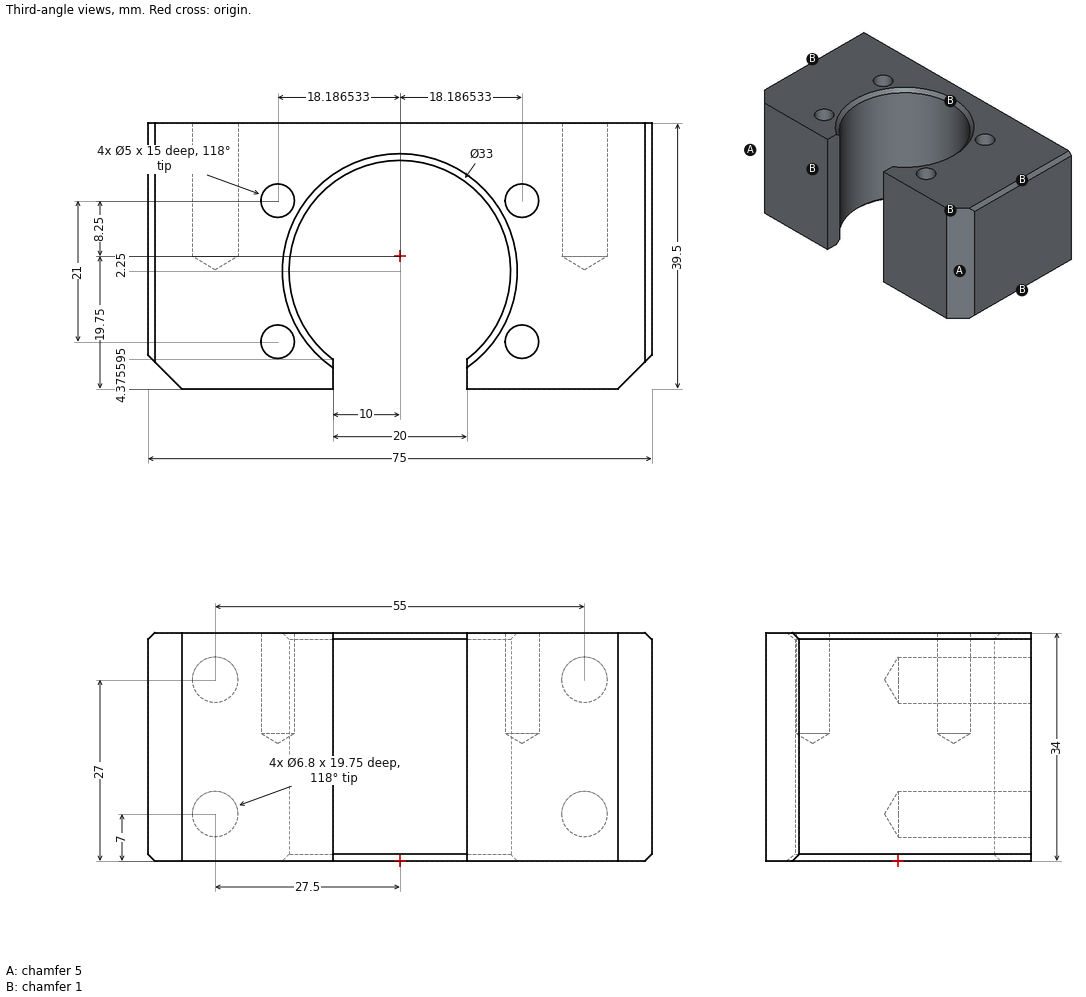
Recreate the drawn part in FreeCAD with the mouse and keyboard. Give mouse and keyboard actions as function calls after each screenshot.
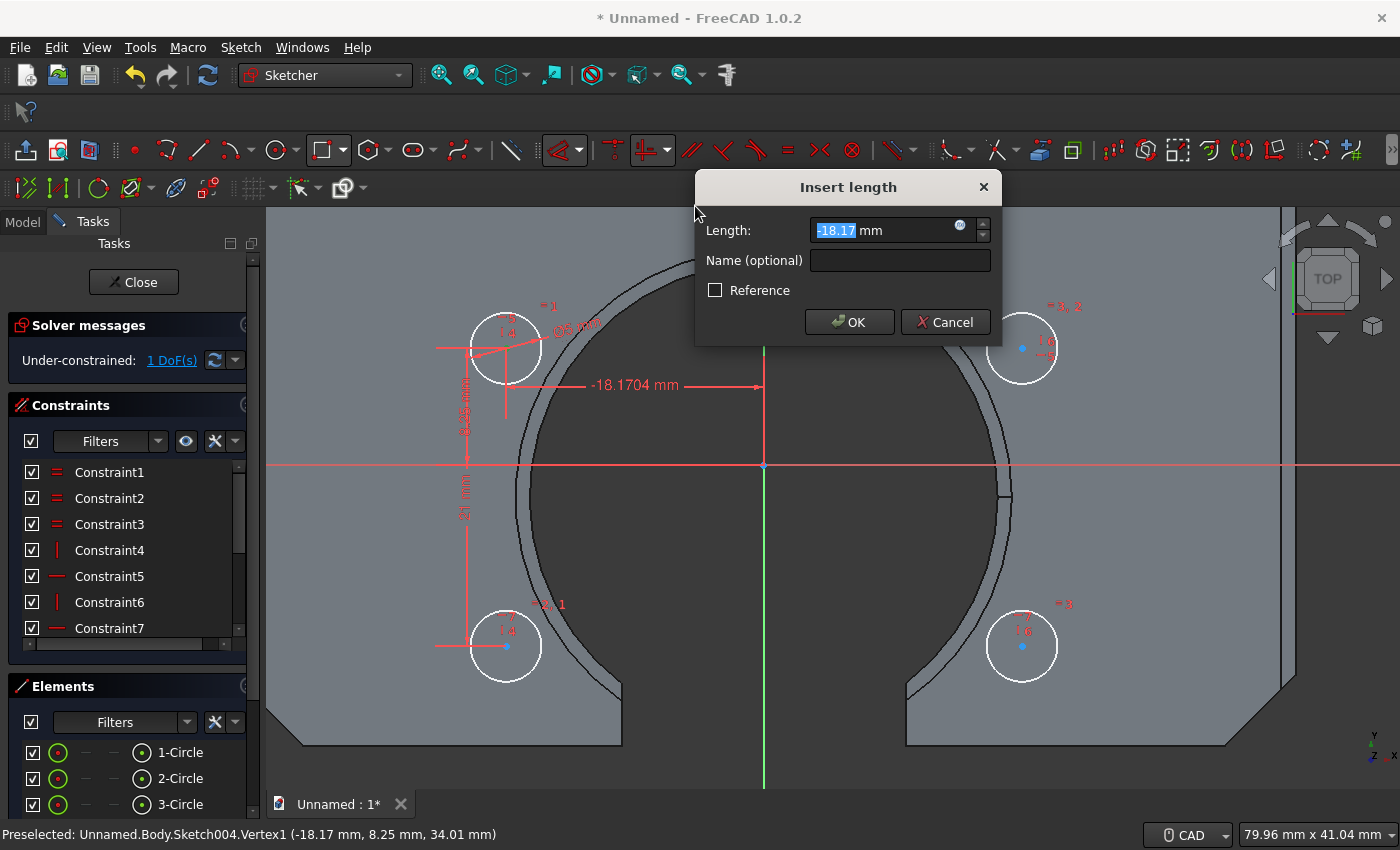
text(-18.186533)
key(Return)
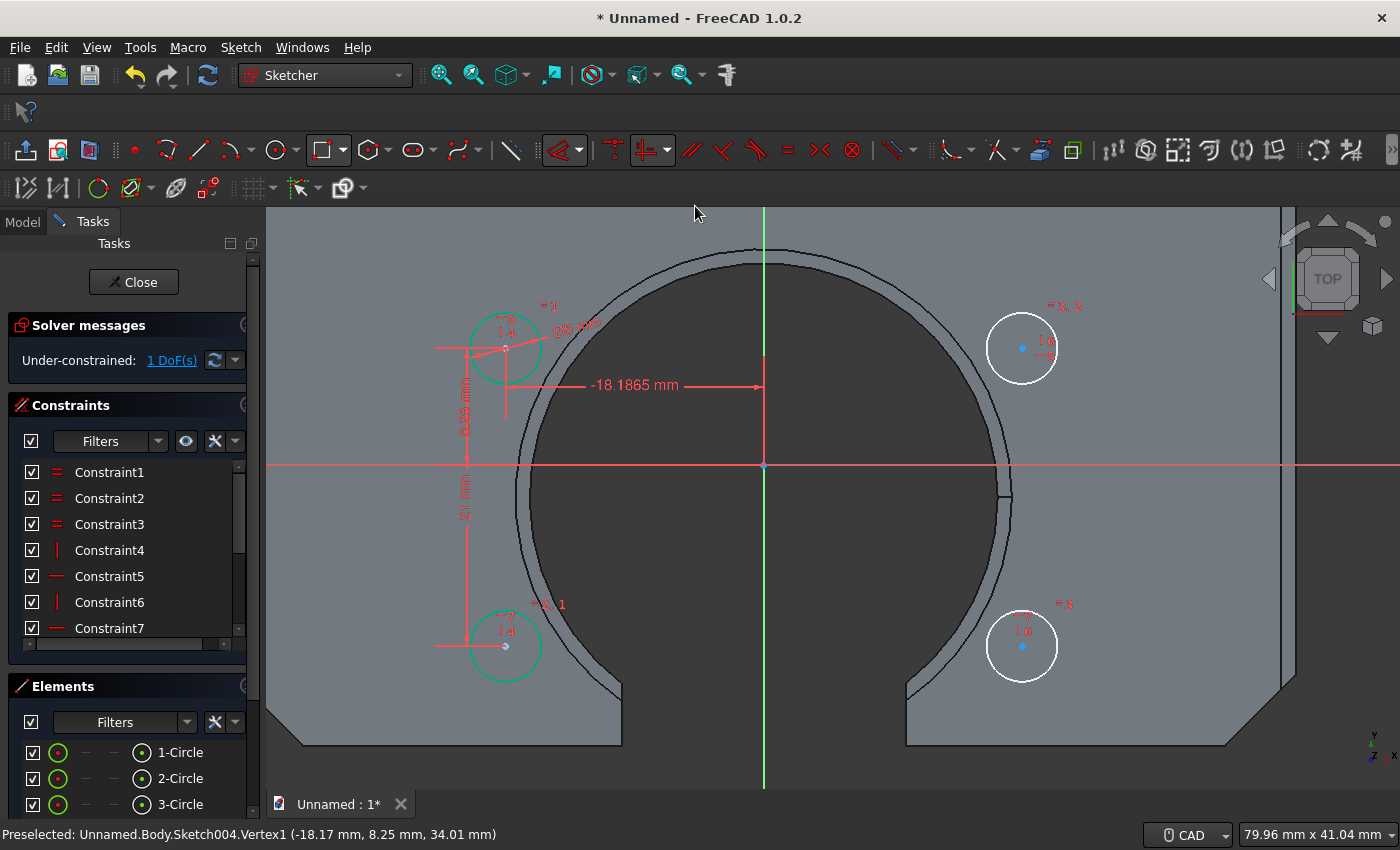
click(1022, 348)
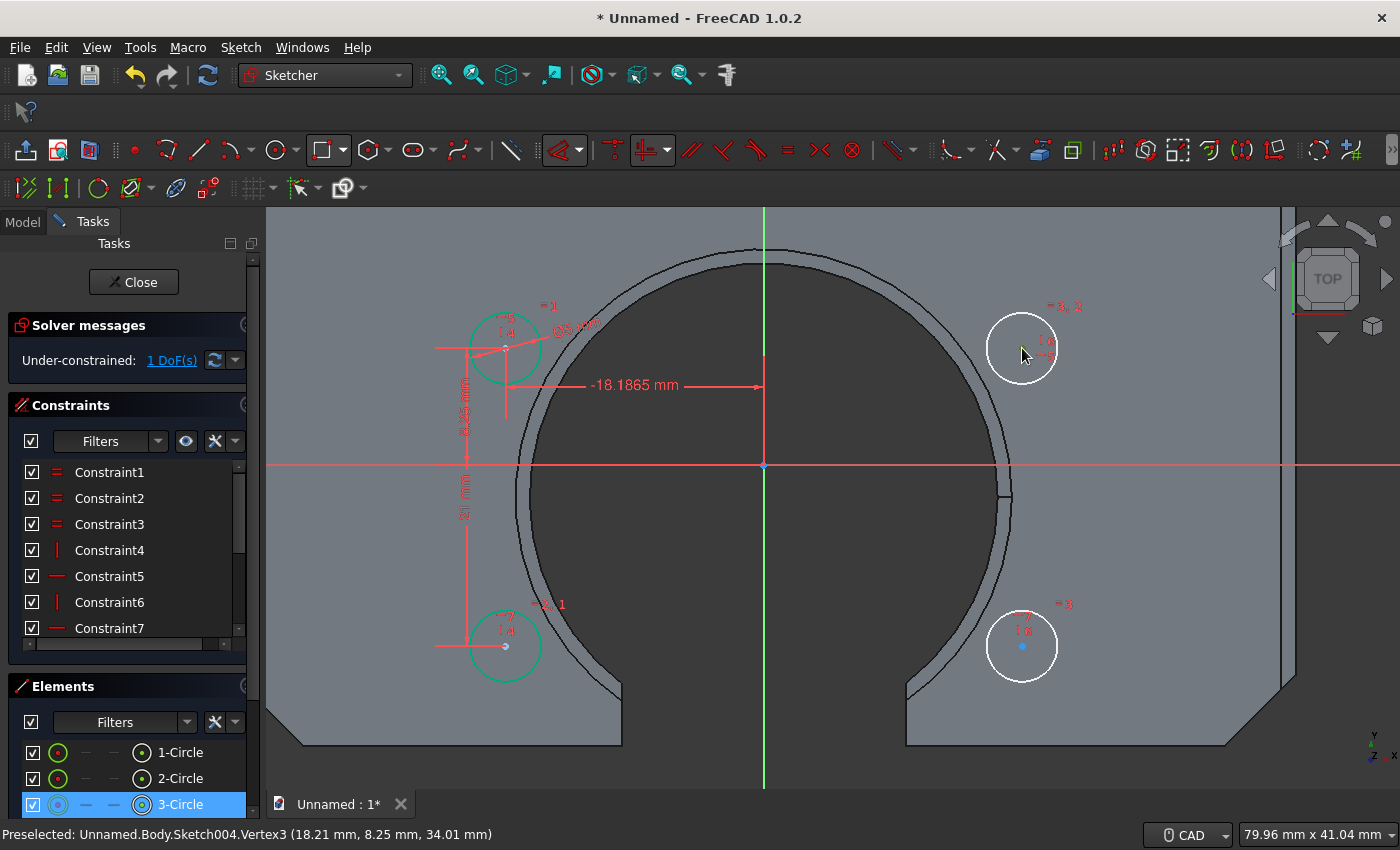
click(582, 150)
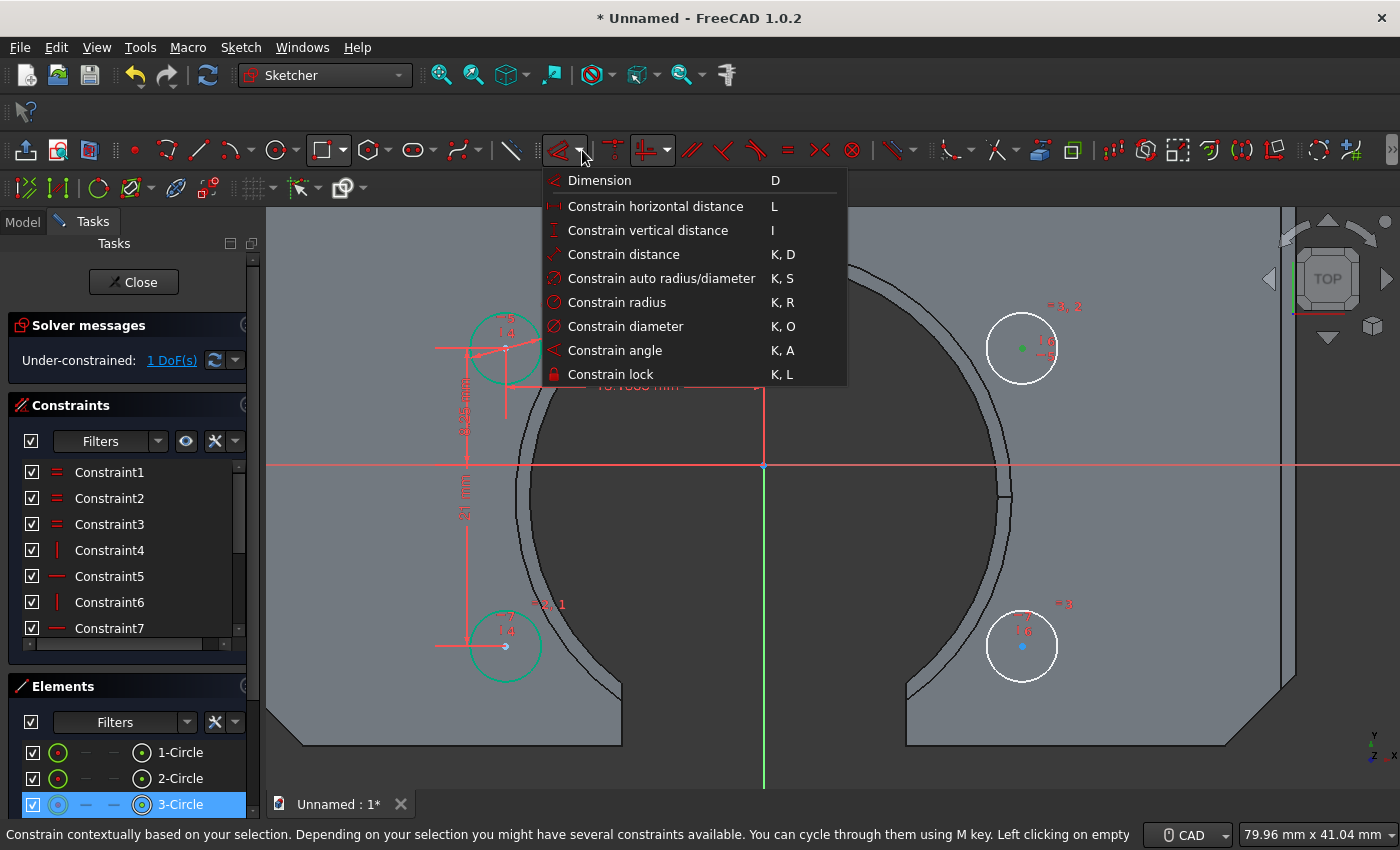
click(695, 206)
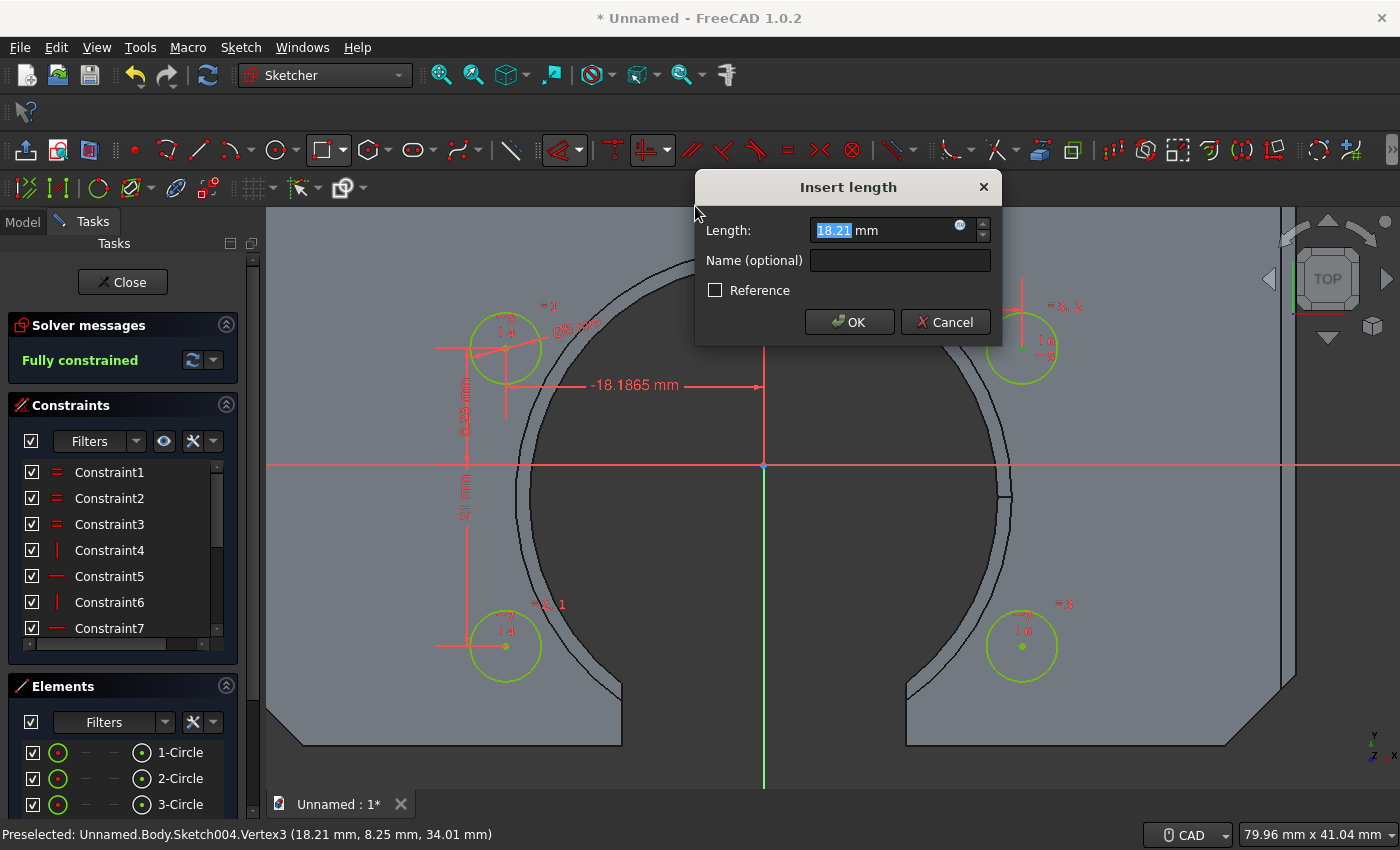
text(18.186533)
key(Return)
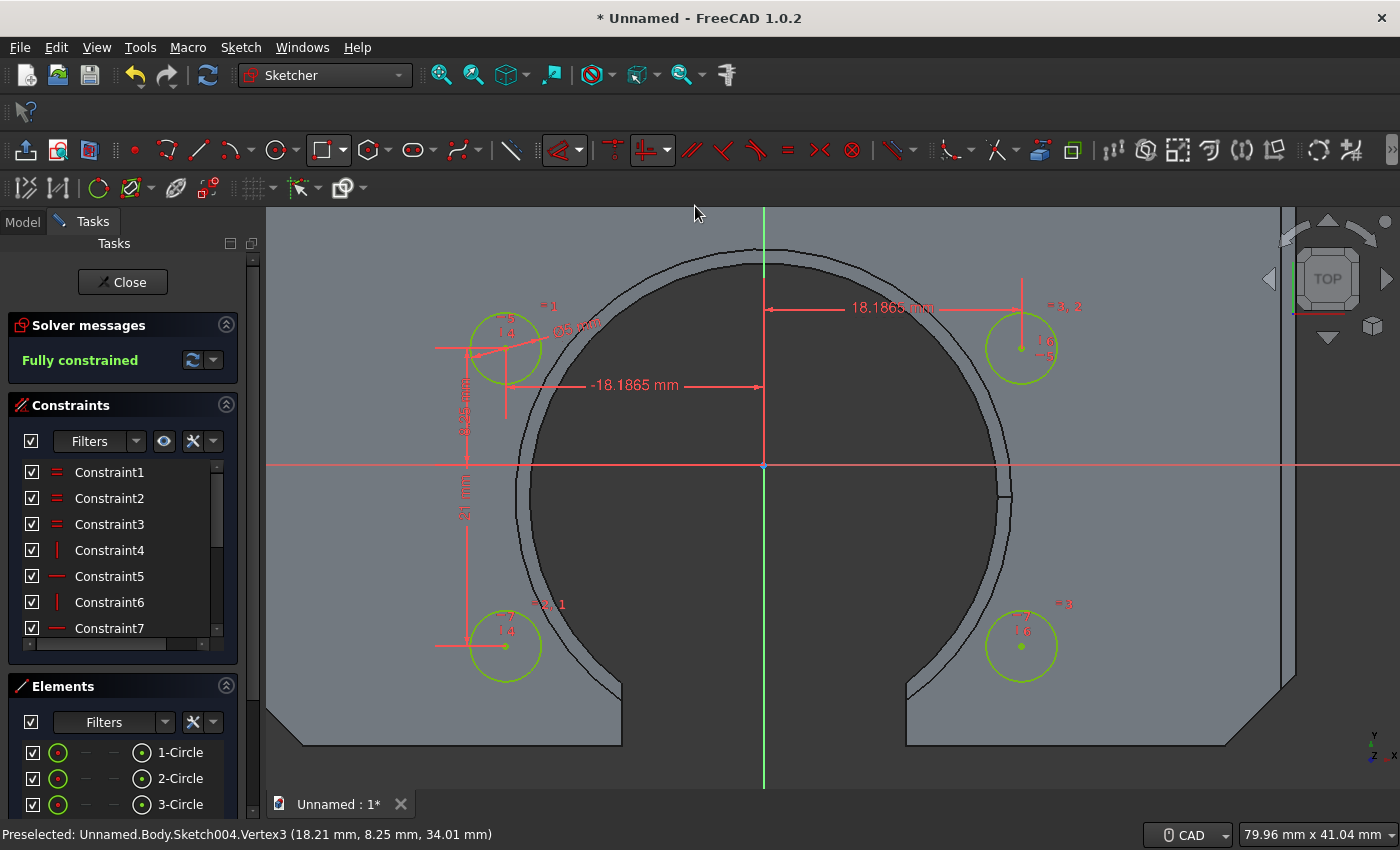
click(123, 282)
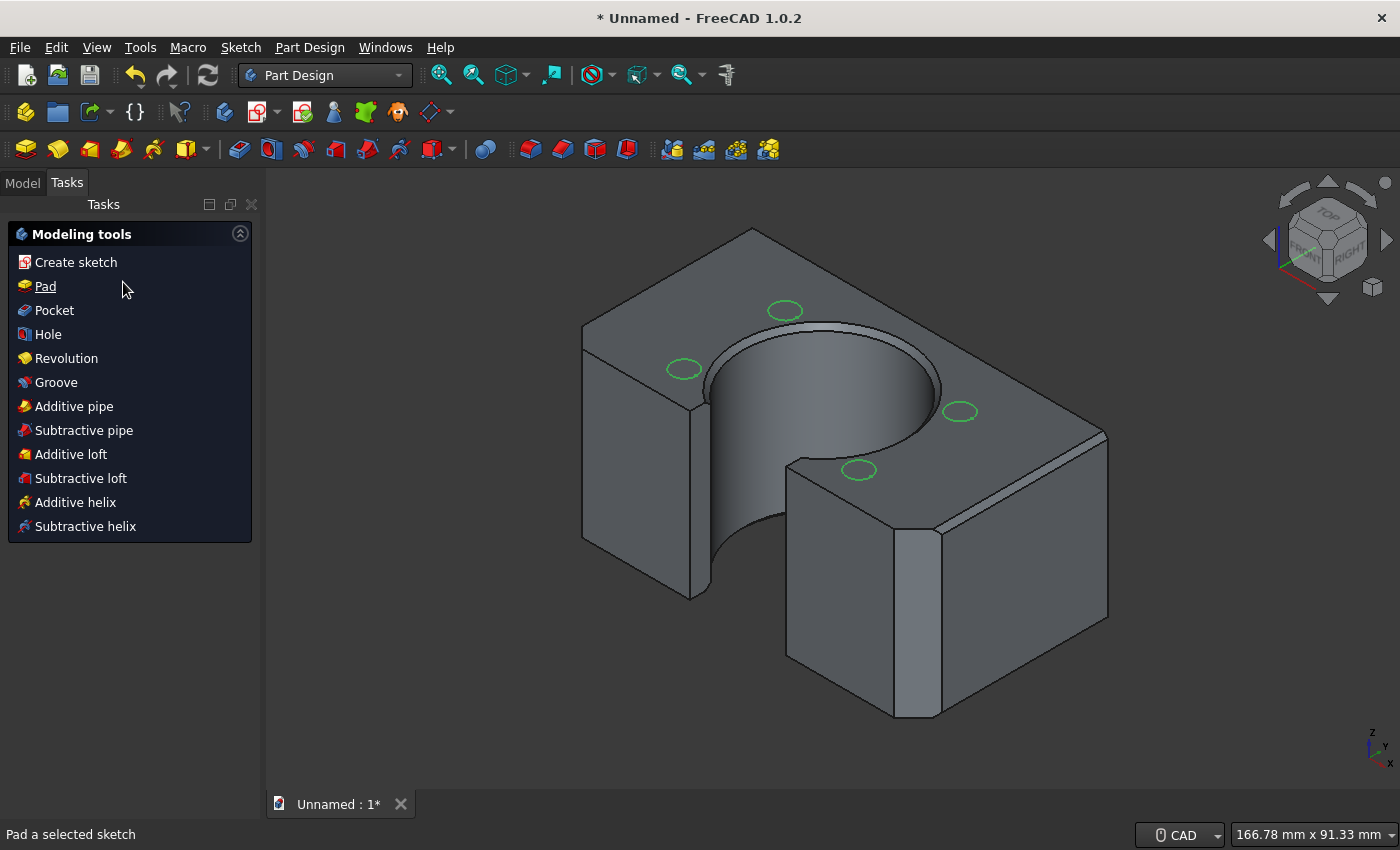
click(272, 150)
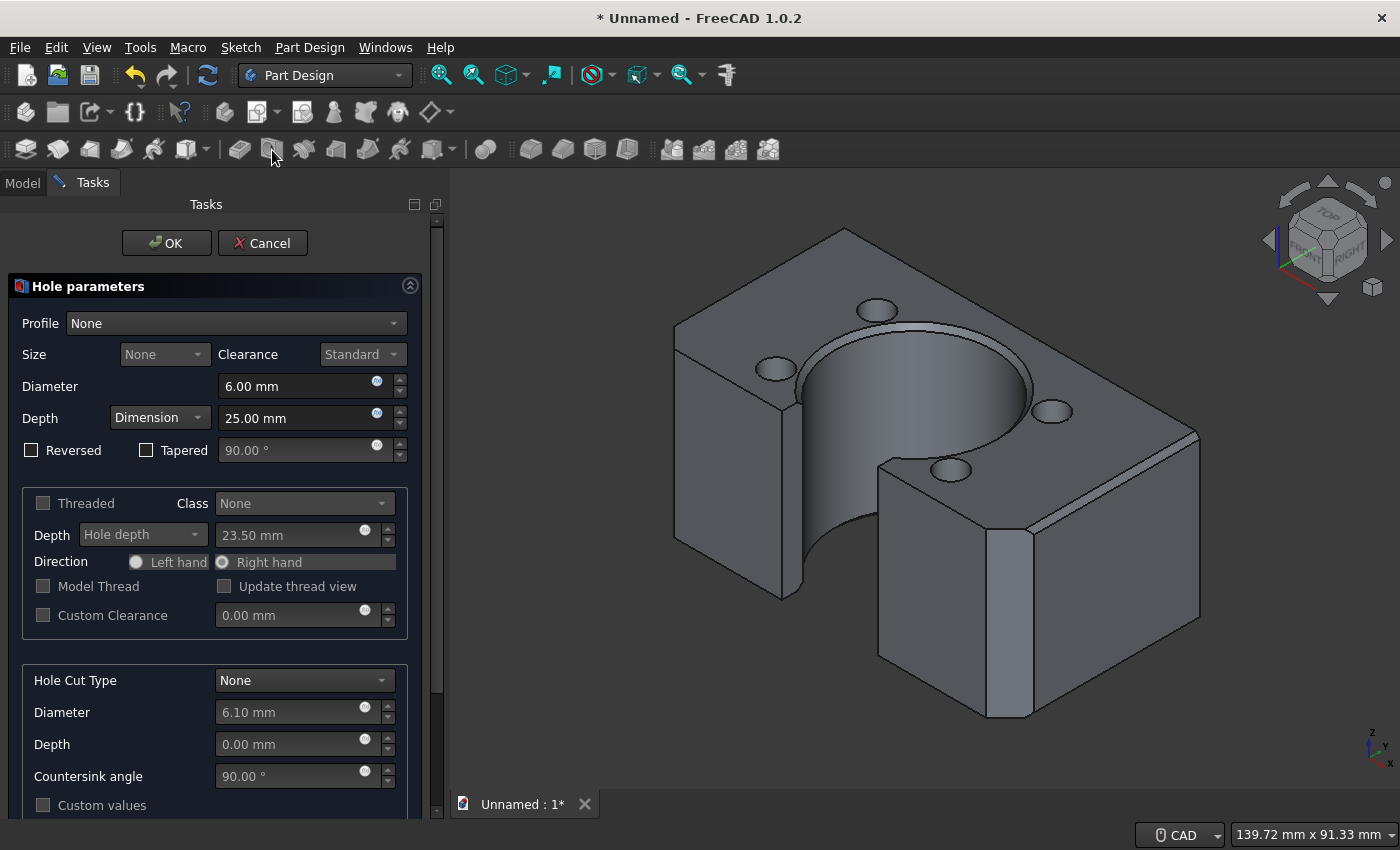
triple_click(305, 386)